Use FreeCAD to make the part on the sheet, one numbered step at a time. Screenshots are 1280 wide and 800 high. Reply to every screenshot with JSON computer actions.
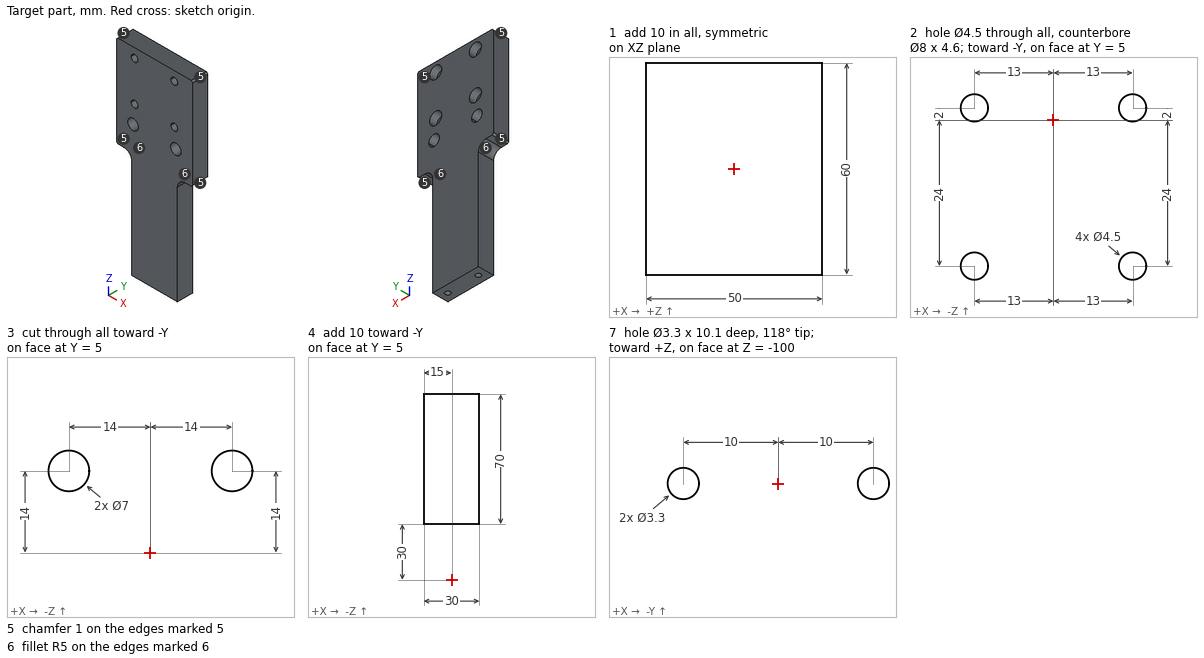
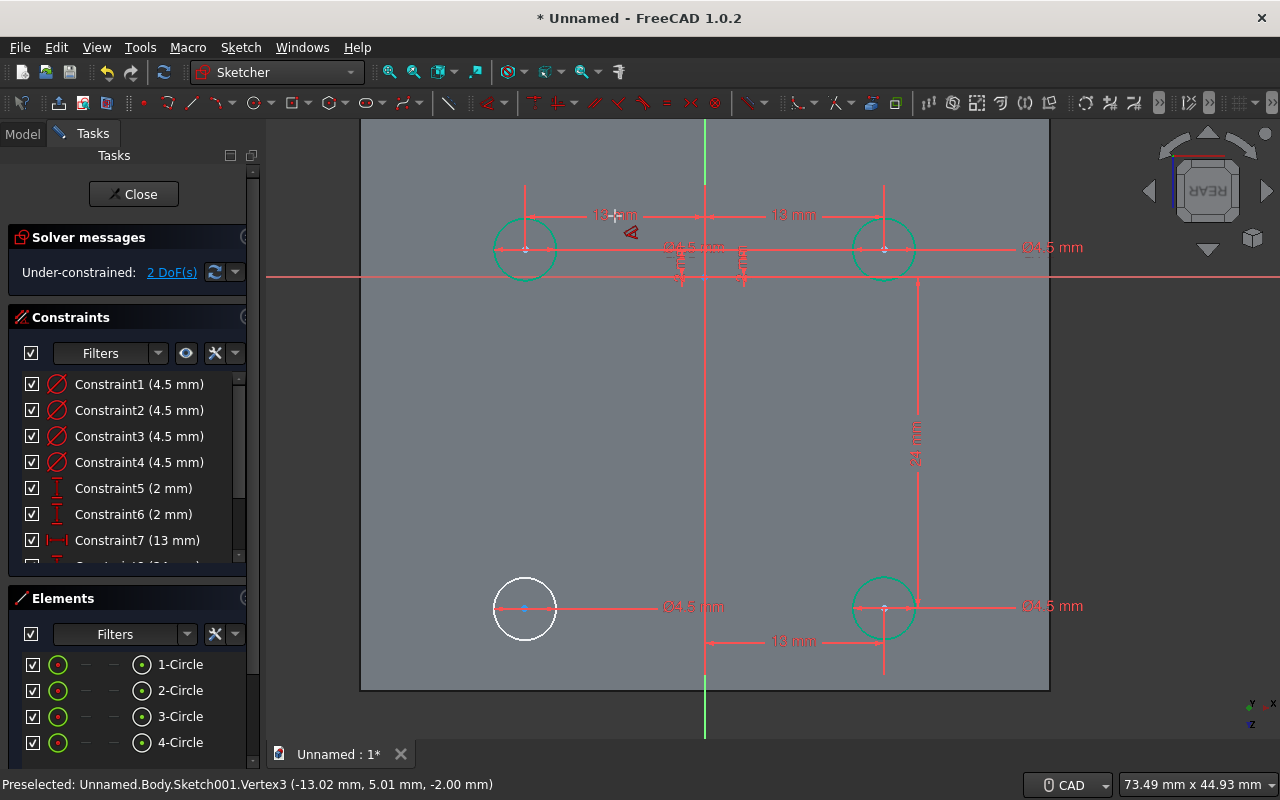
{"action": "left_click", "coordinate": [525, 609]}
{"action": "left_click", "coordinate": [615, 643]}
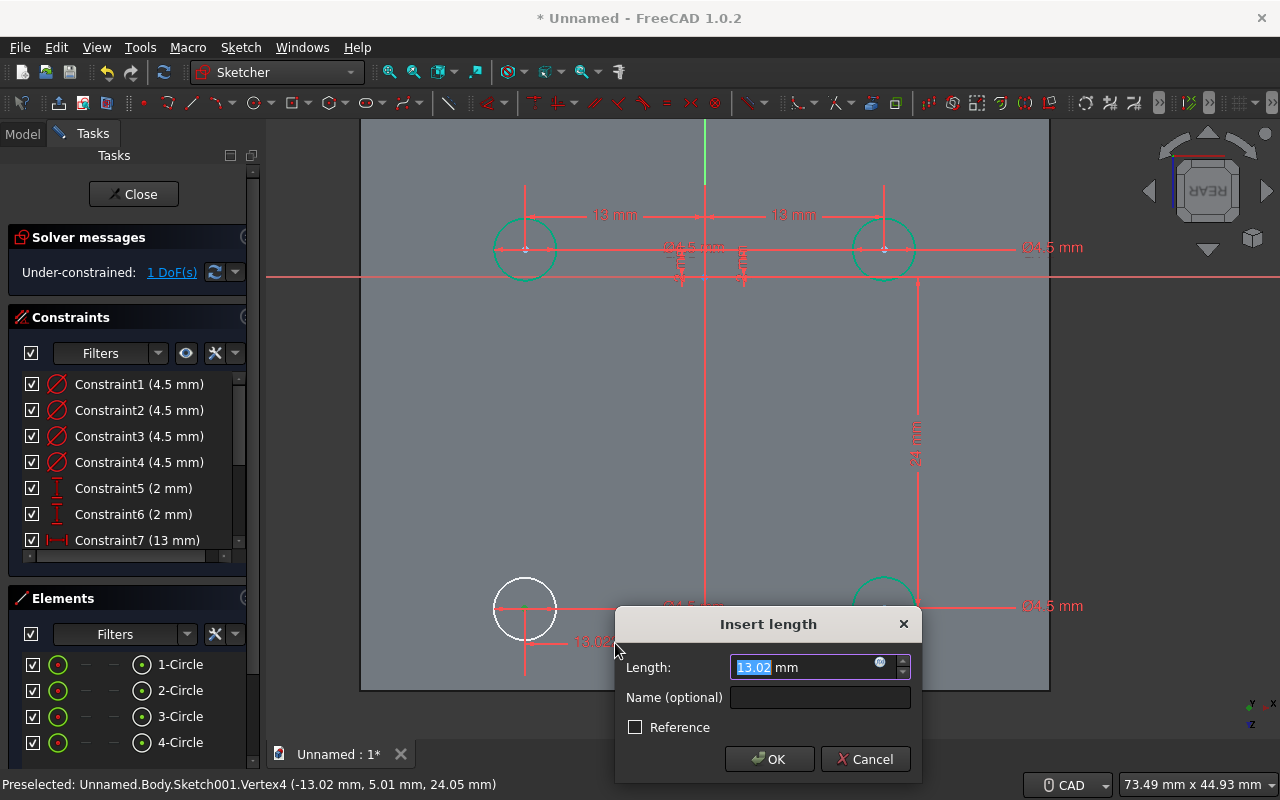
{"action": "type", "text": "13"}
{"action": "key", "text": "Return"}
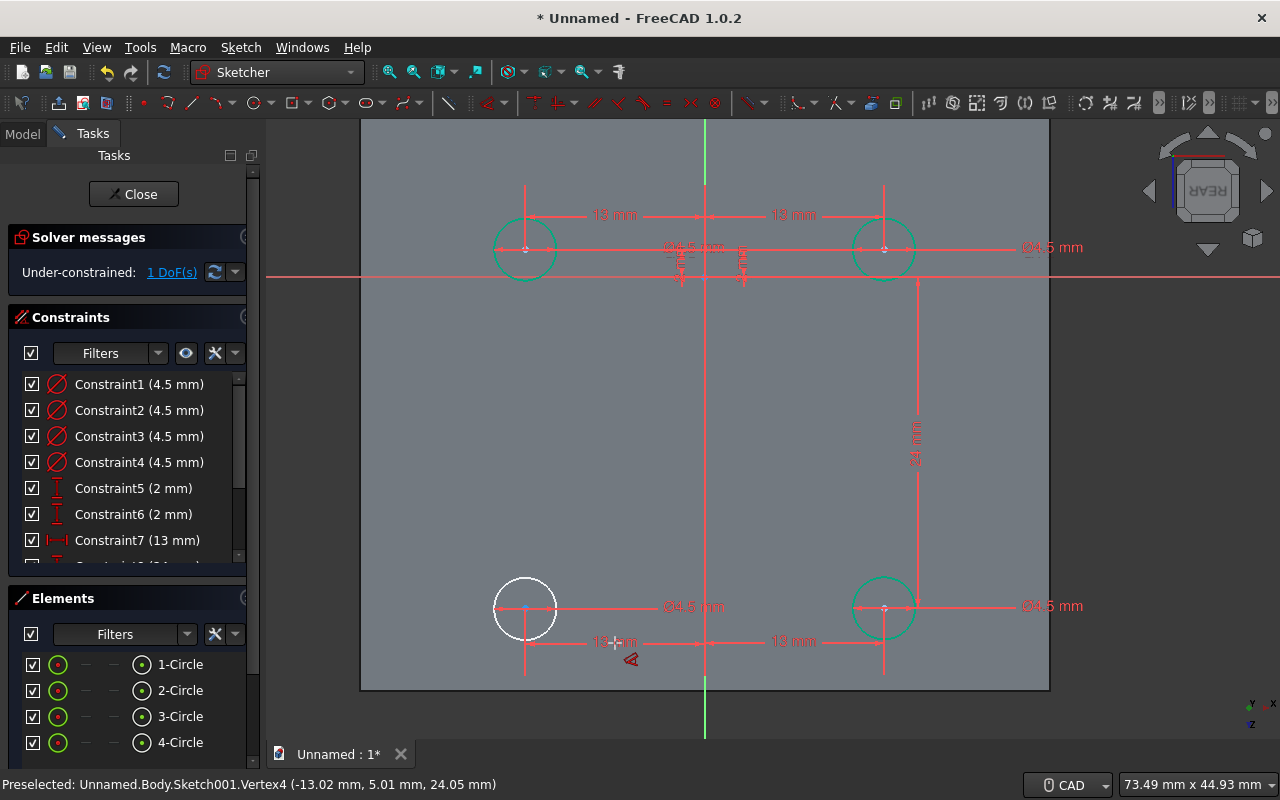
{"action": "left_click", "coordinate": [525, 609]}
{"action": "left_click", "coordinate": [491, 443]}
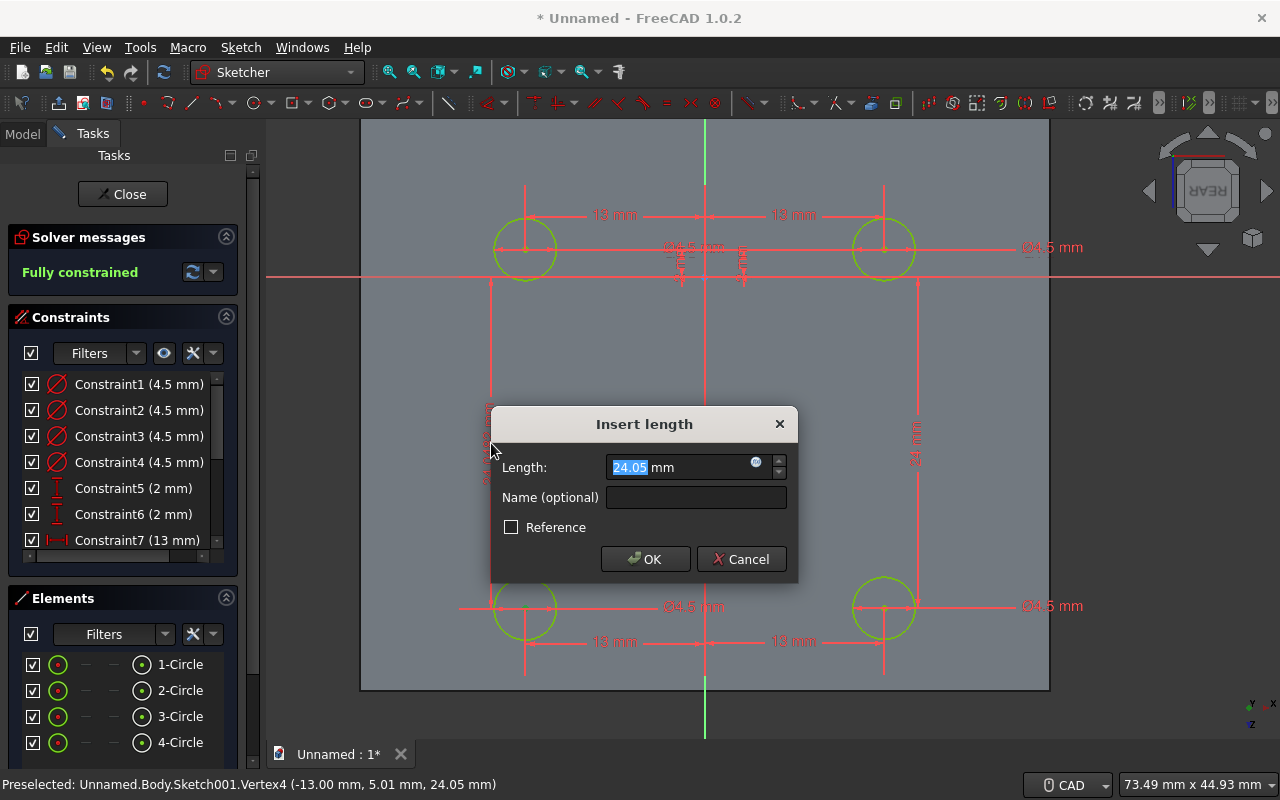
{"action": "type", "text": "24"}
{"action": "key", "text": "Return"}
{"action": "key", "text": "Escape"}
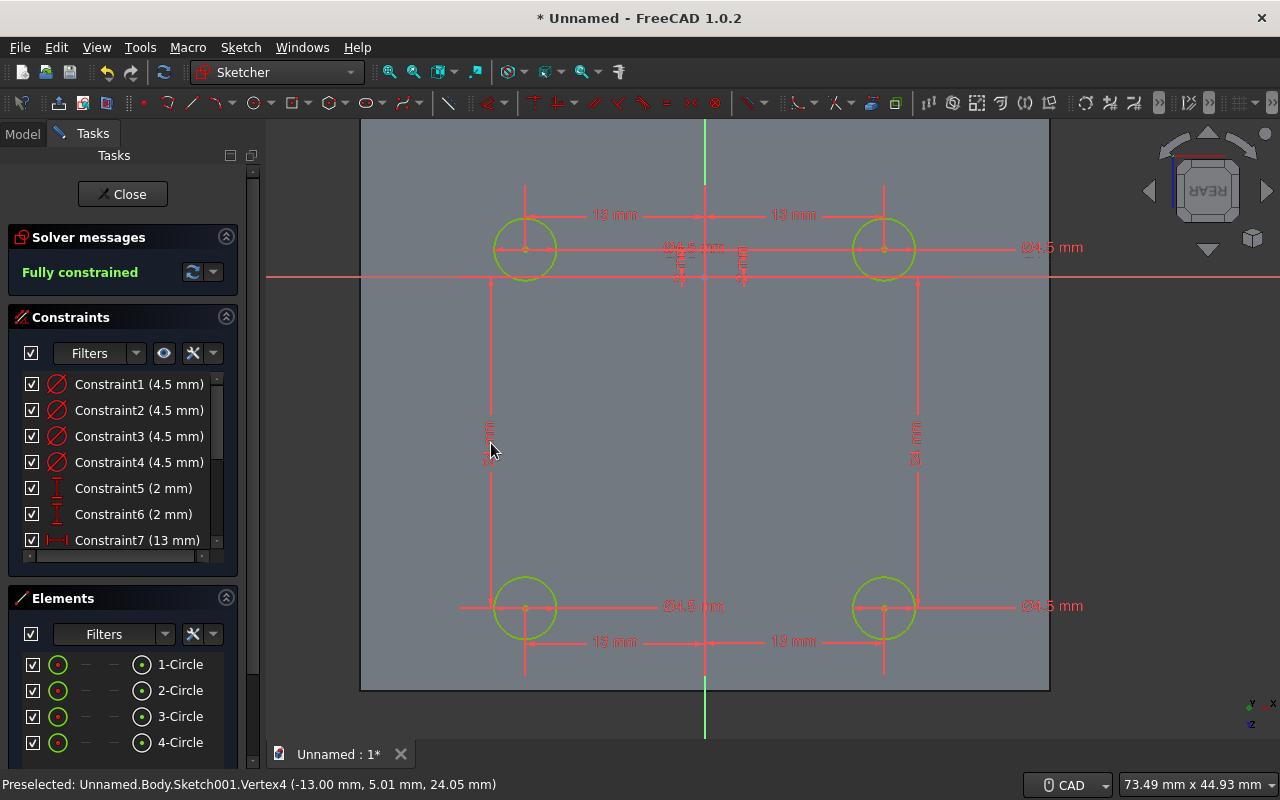
{"action": "left_click", "coordinate": [123, 194]}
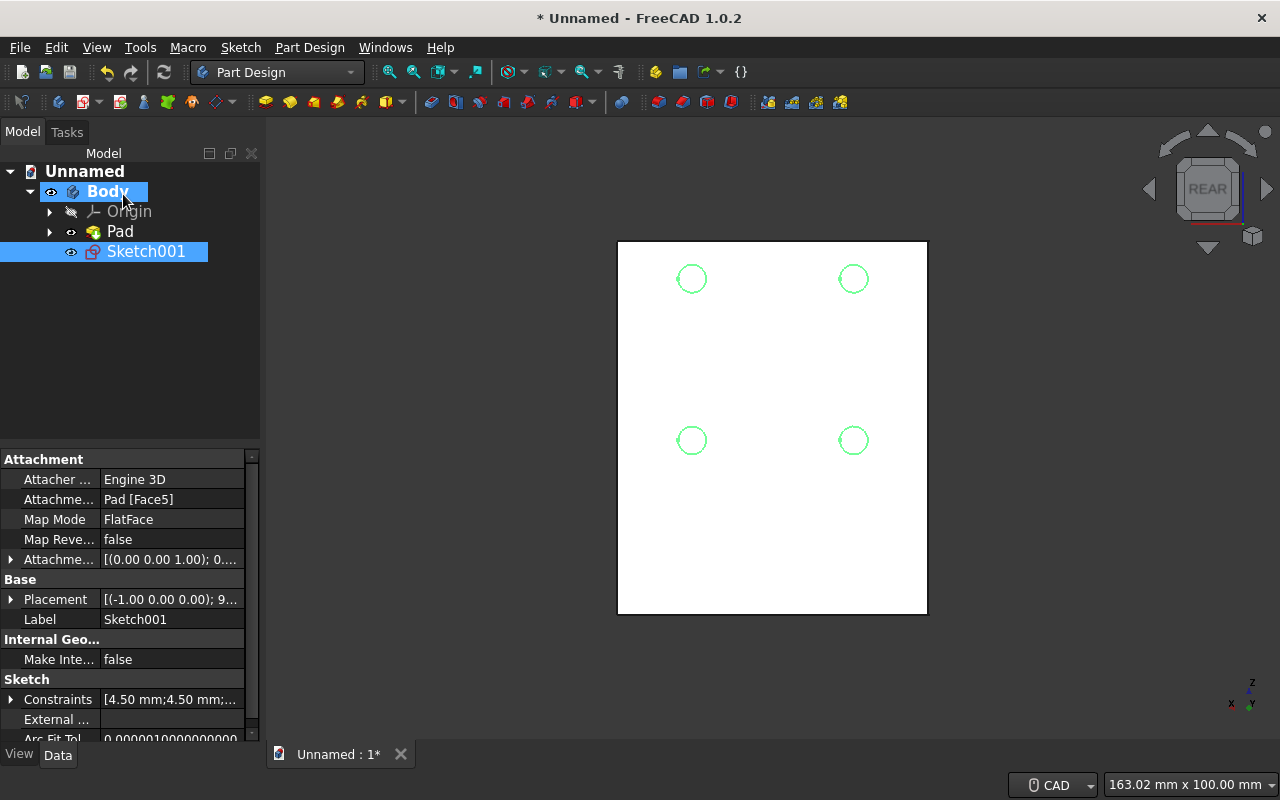
{"action": "left_click", "coordinate": [456, 102]}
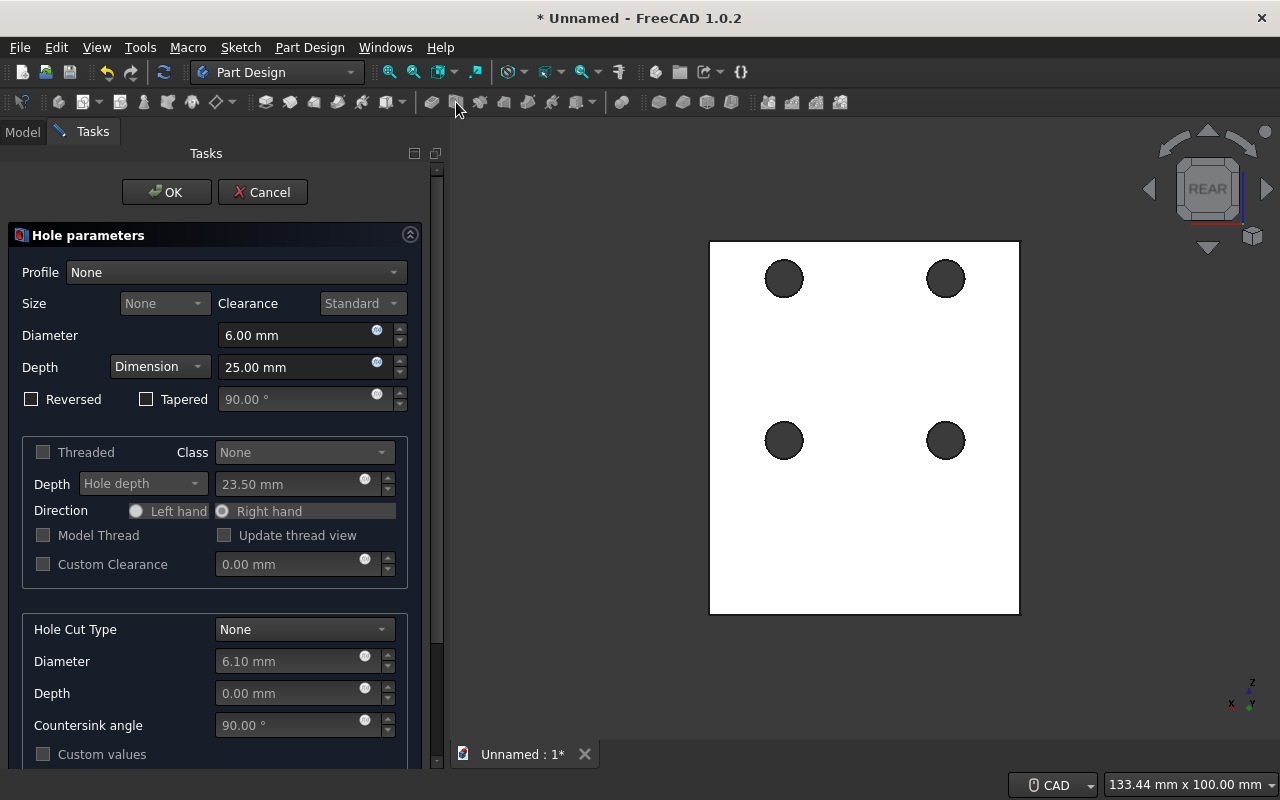
{"action": "triple_click", "coordinate": [305, 335]}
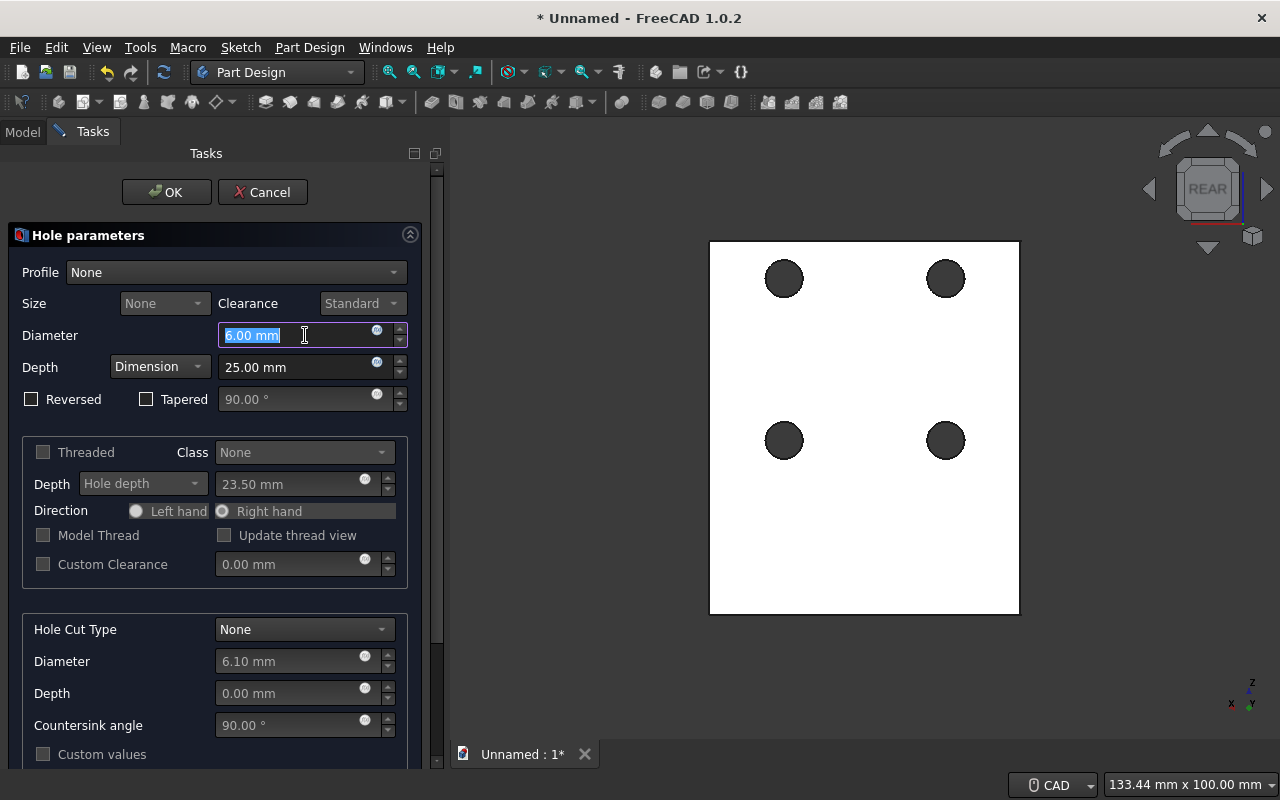
{"action": "type", "text": "4.5"}
{"action": "key", "text": "Tab"}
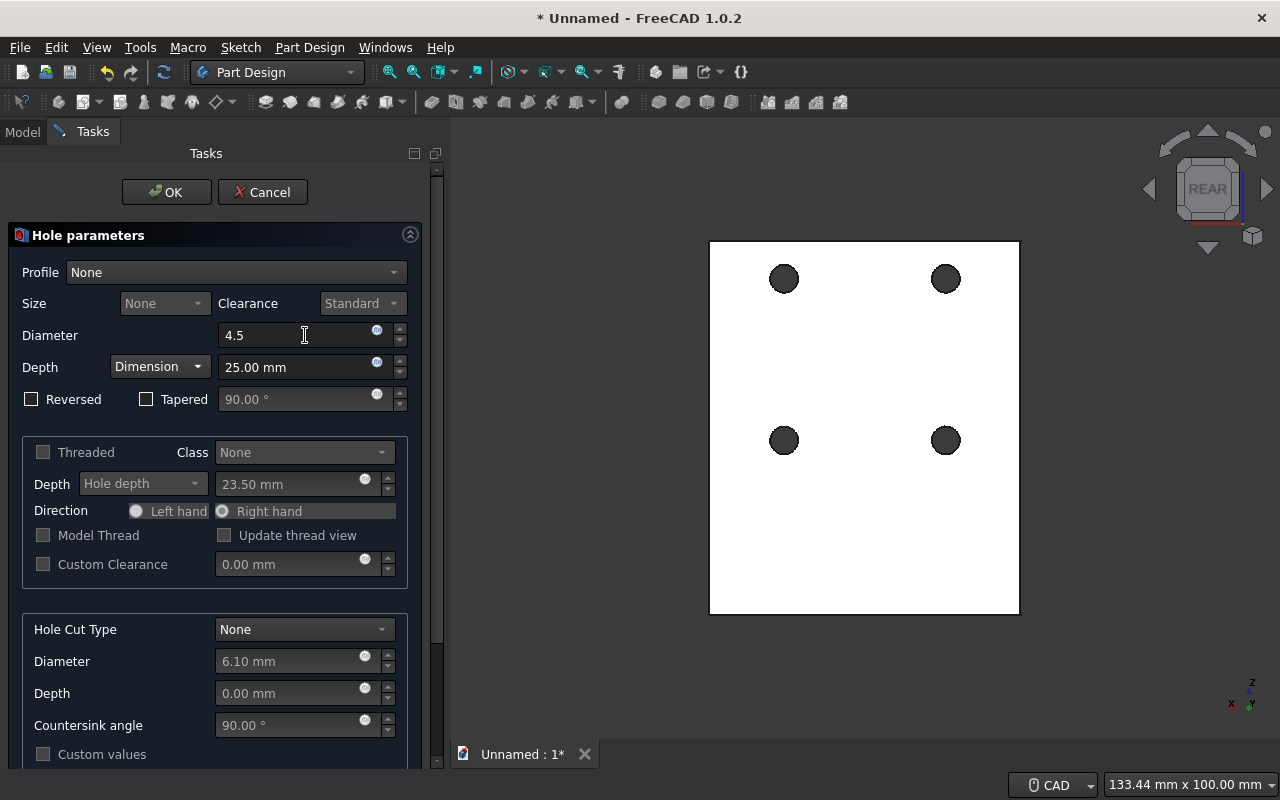
{"action": "left_click", "coordinate": [161, 366]}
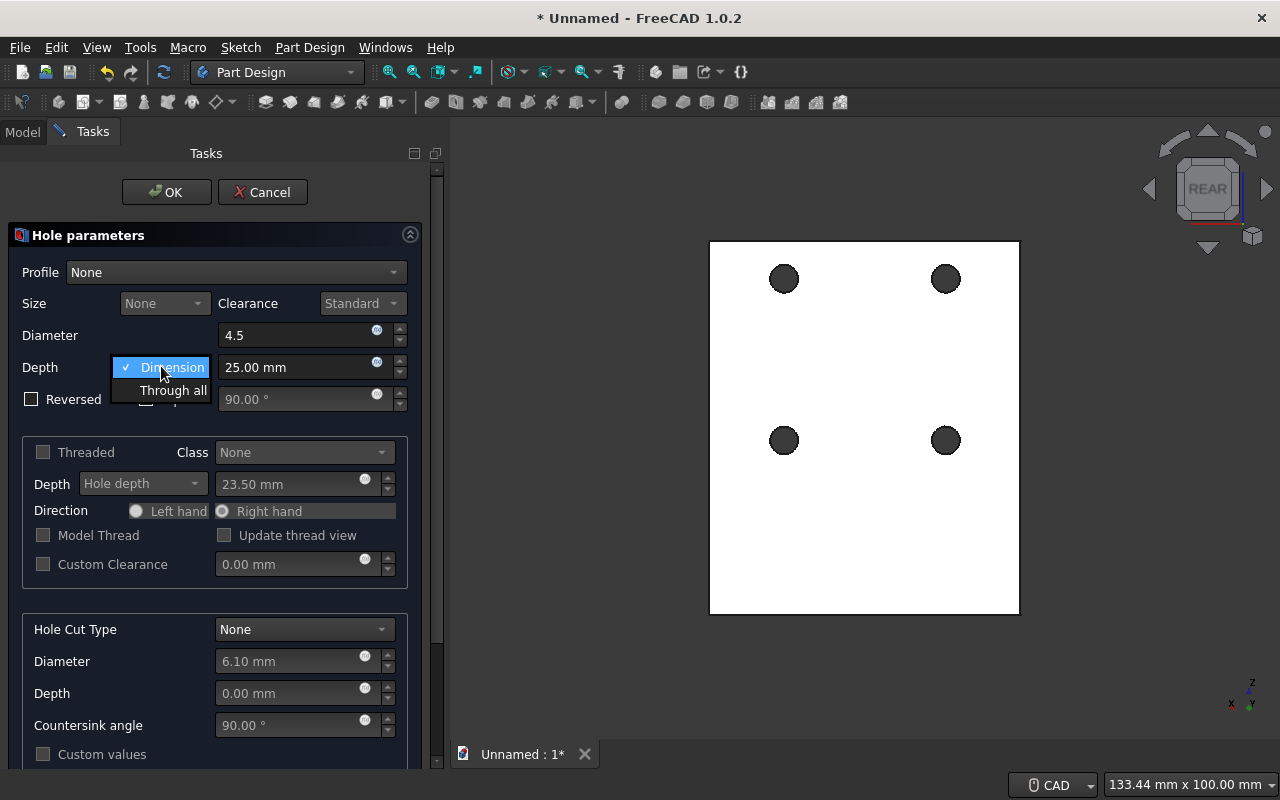
{"action": "left_click", "coordinate": [160, 390]}